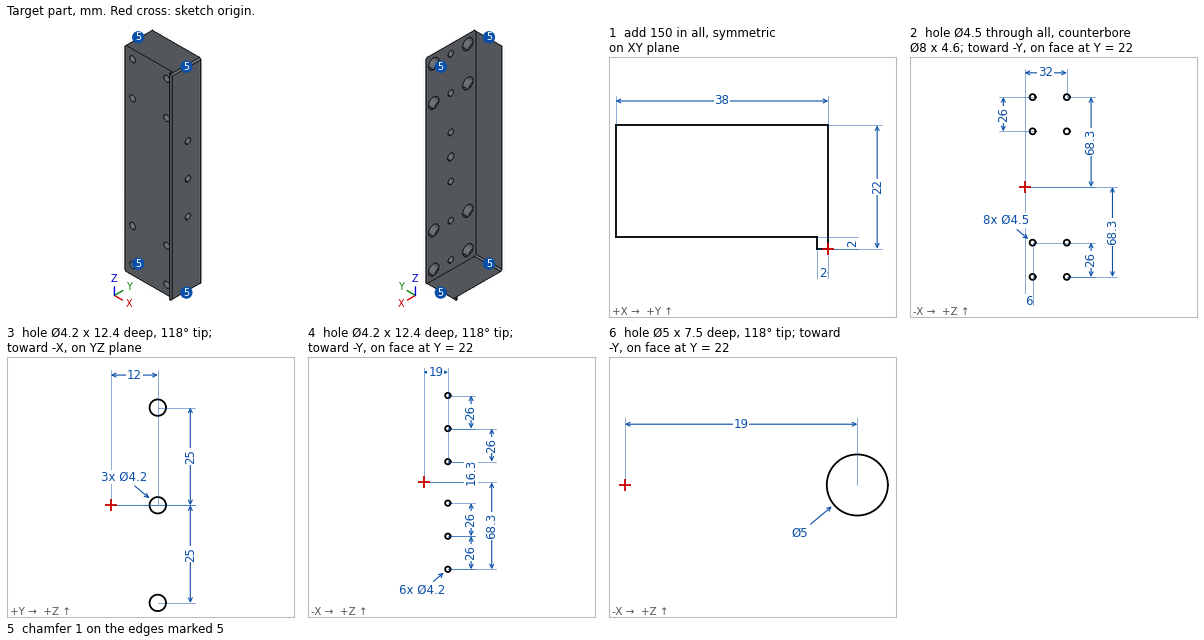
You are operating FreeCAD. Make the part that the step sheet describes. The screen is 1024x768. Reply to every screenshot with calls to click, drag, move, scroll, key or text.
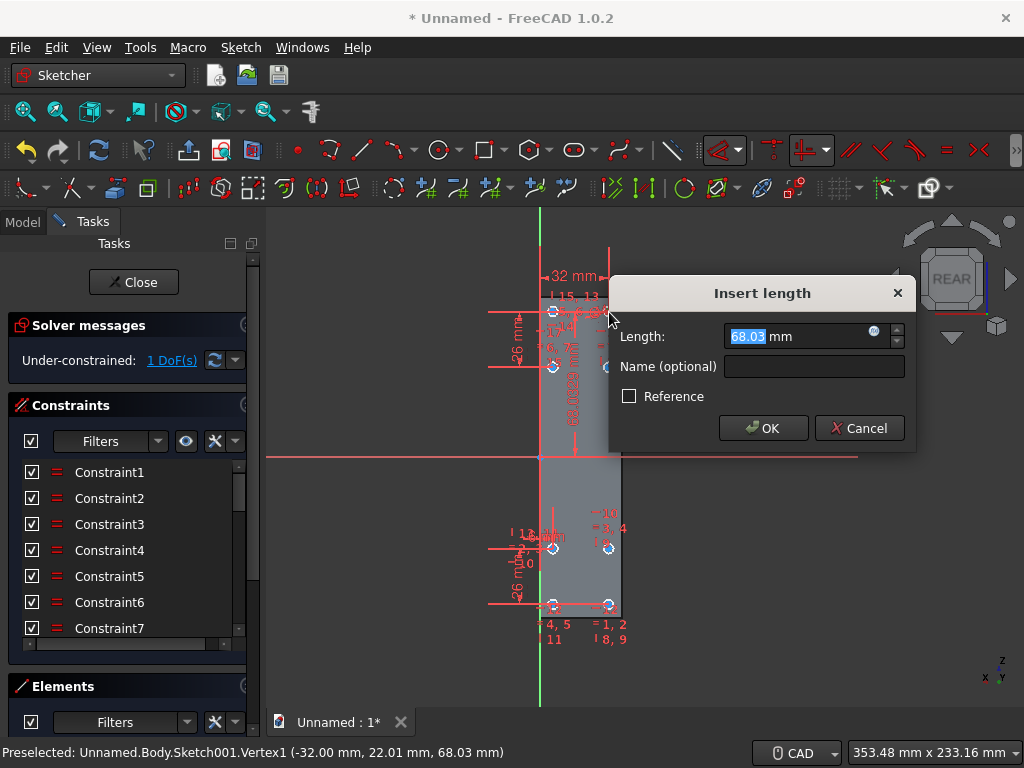
text(68.3)
key(Return)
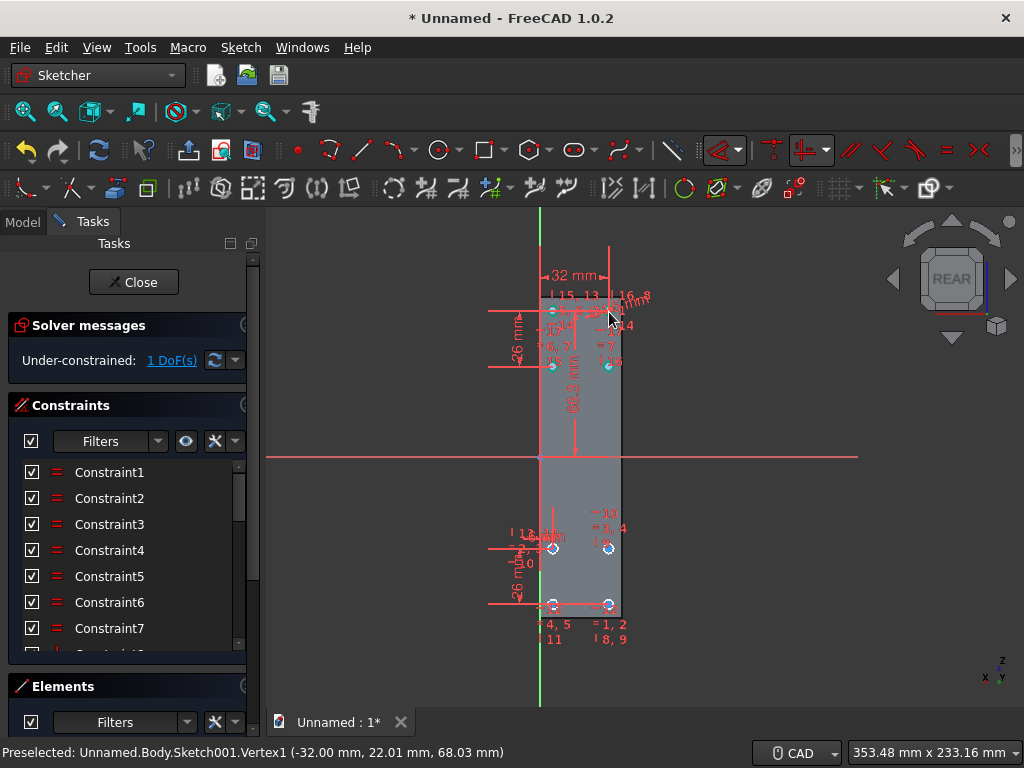
click(609, 604)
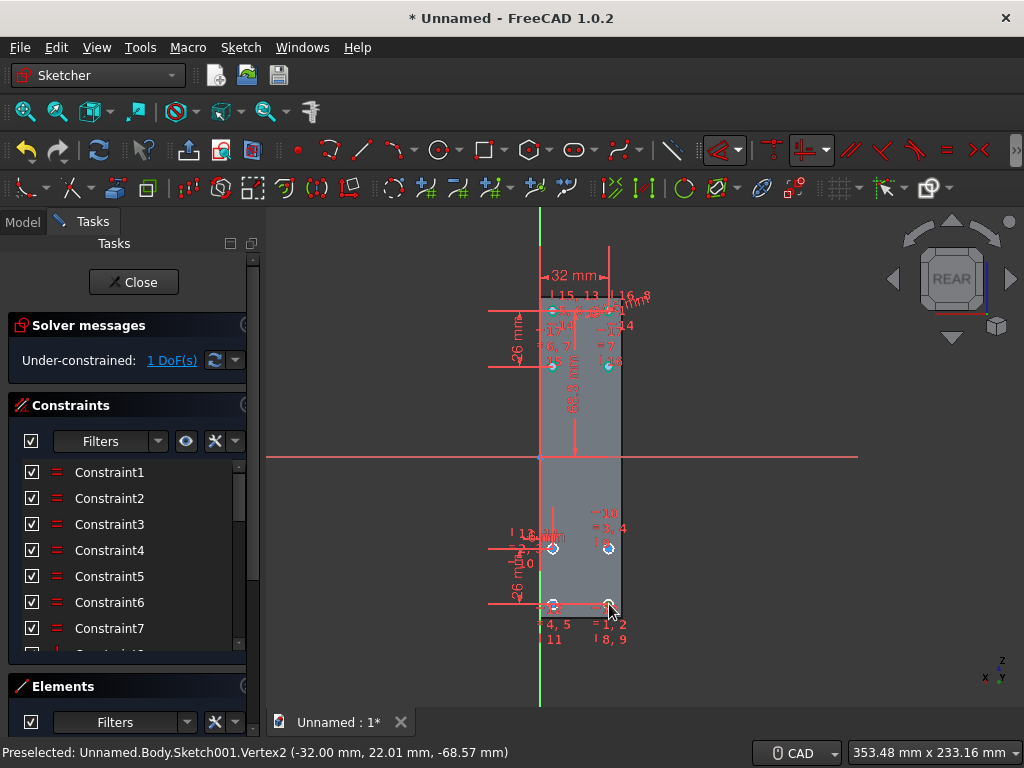
key(i)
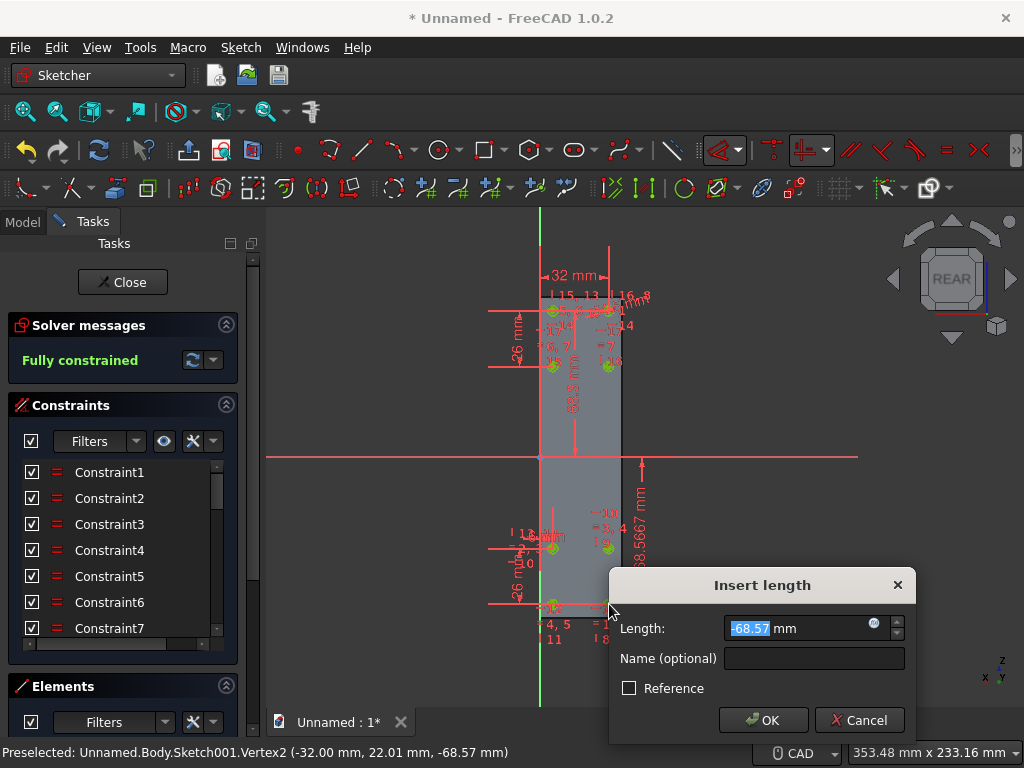
text(-68.3)
key(Return)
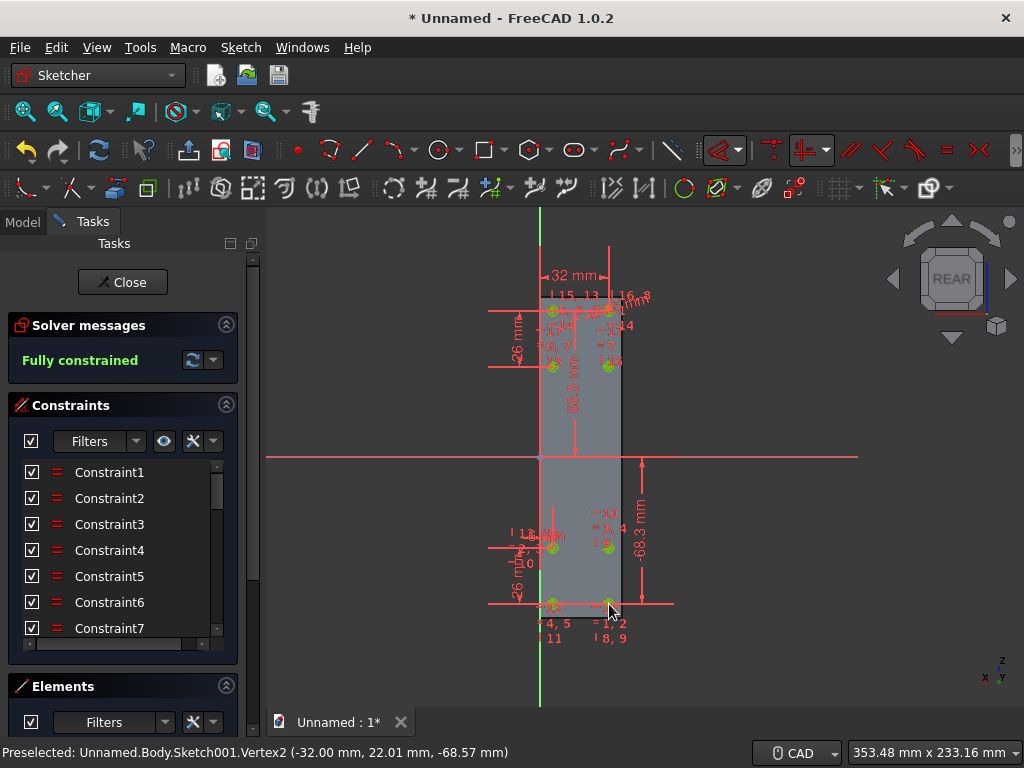
click(123, 282)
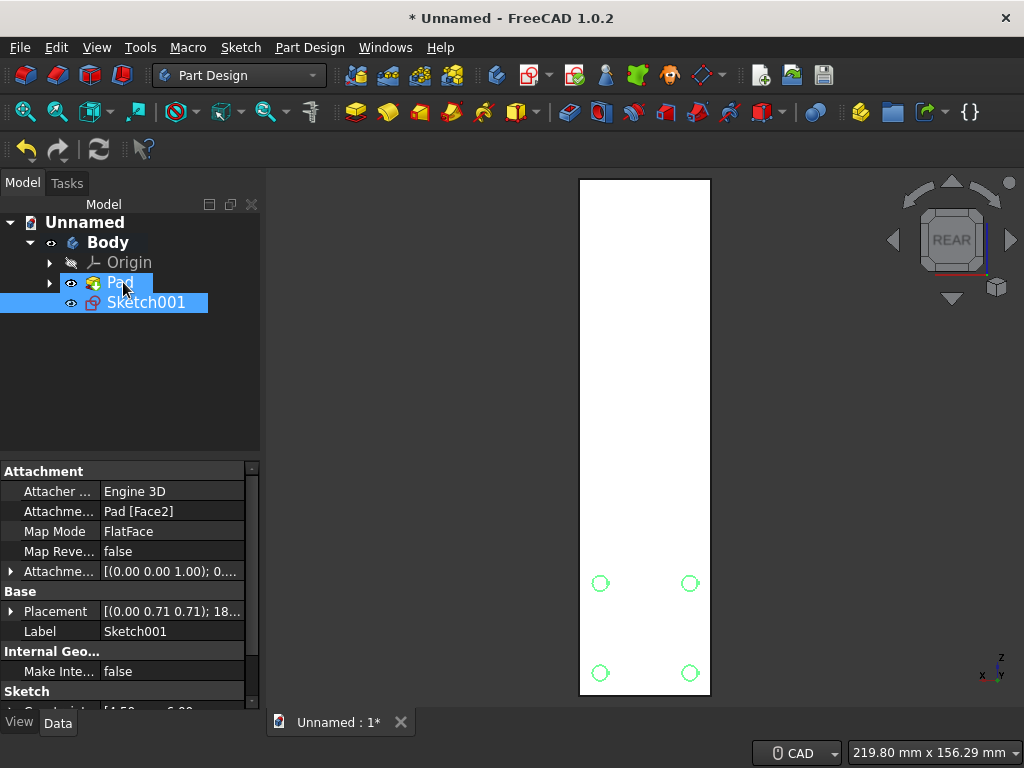
click(602, 112)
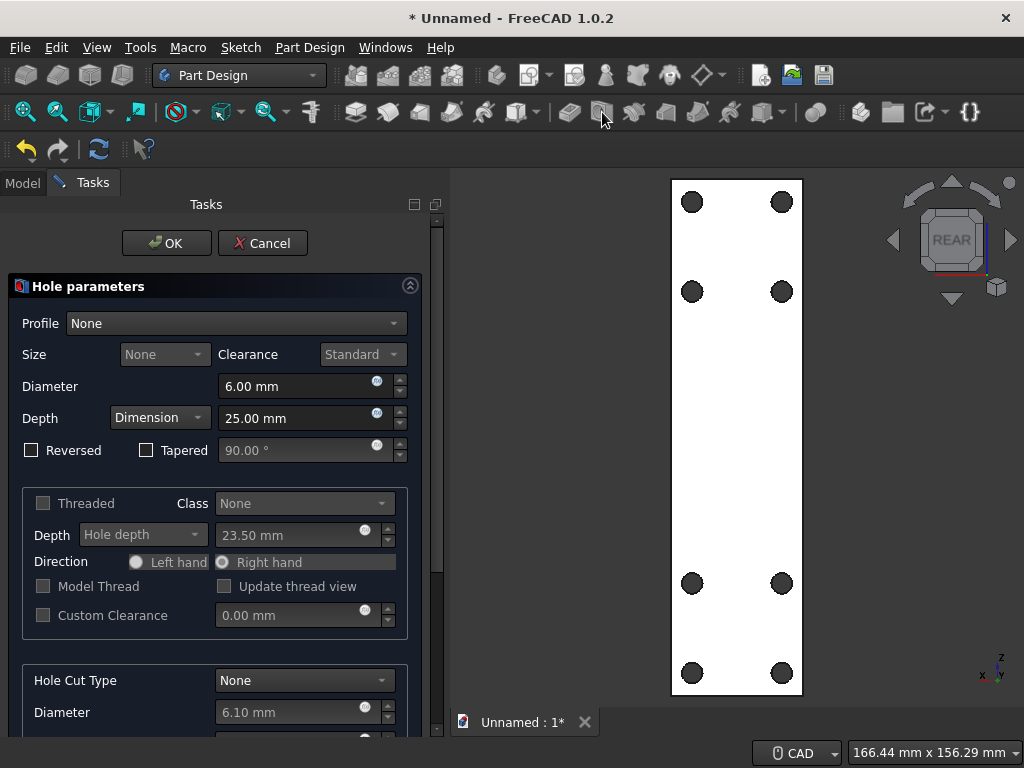
triple_click(305, 386)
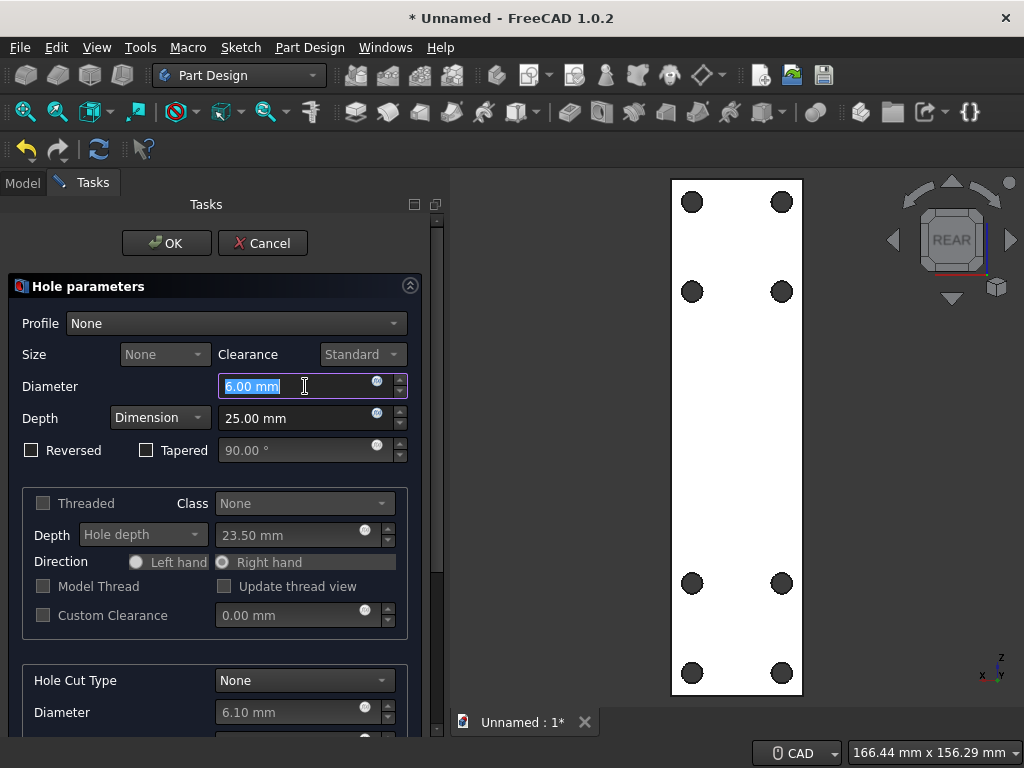
text(4.5)
key(Tab)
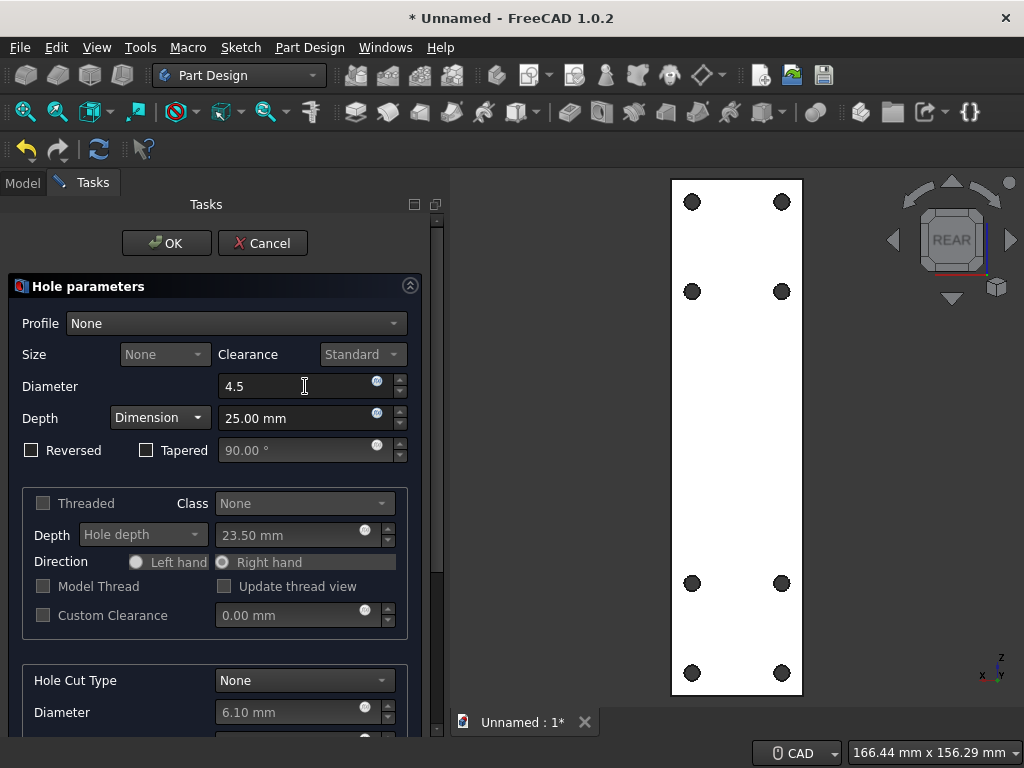
click(161, 418)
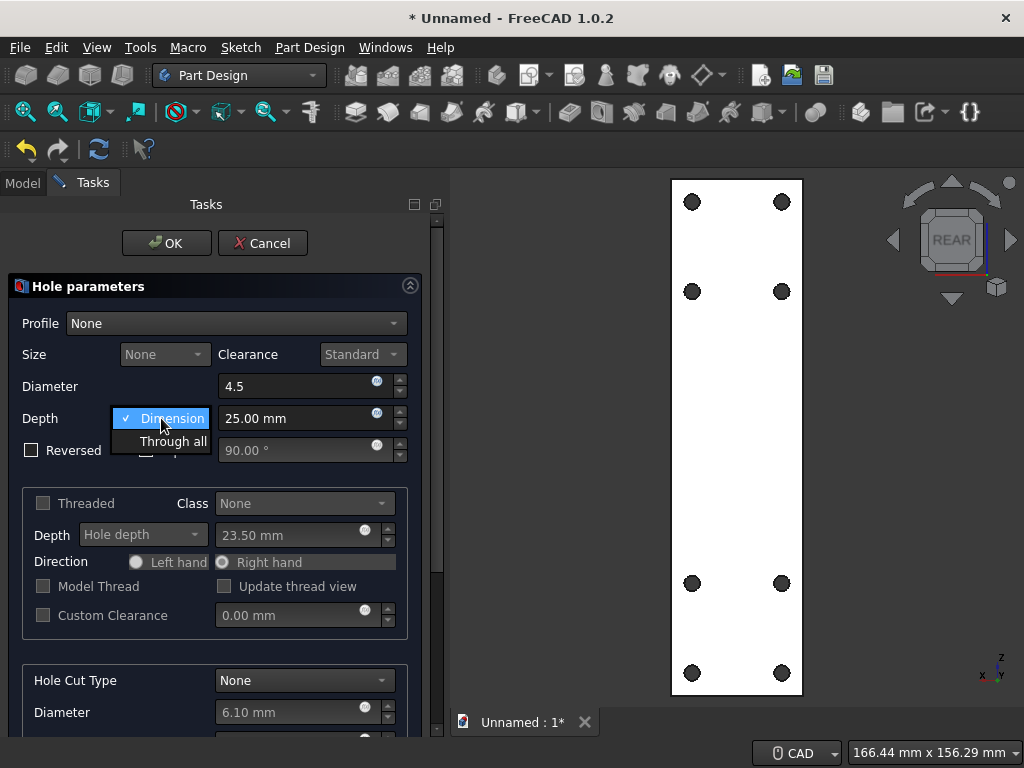
click(160, 442)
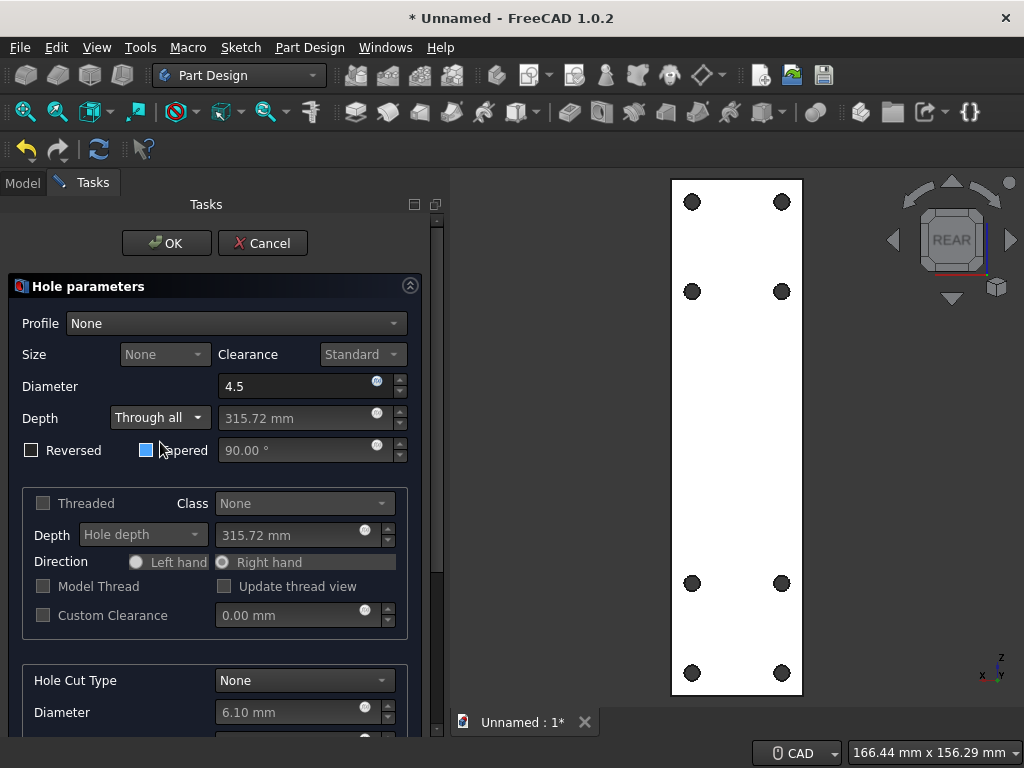
click(306, 680)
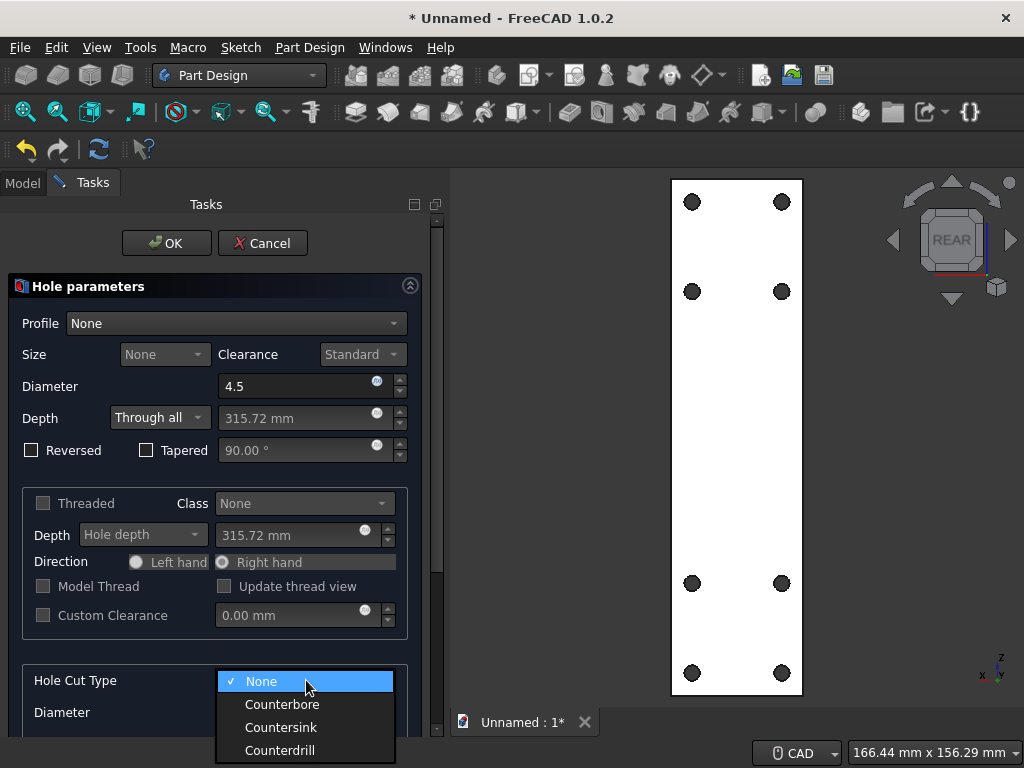
click(304, 704)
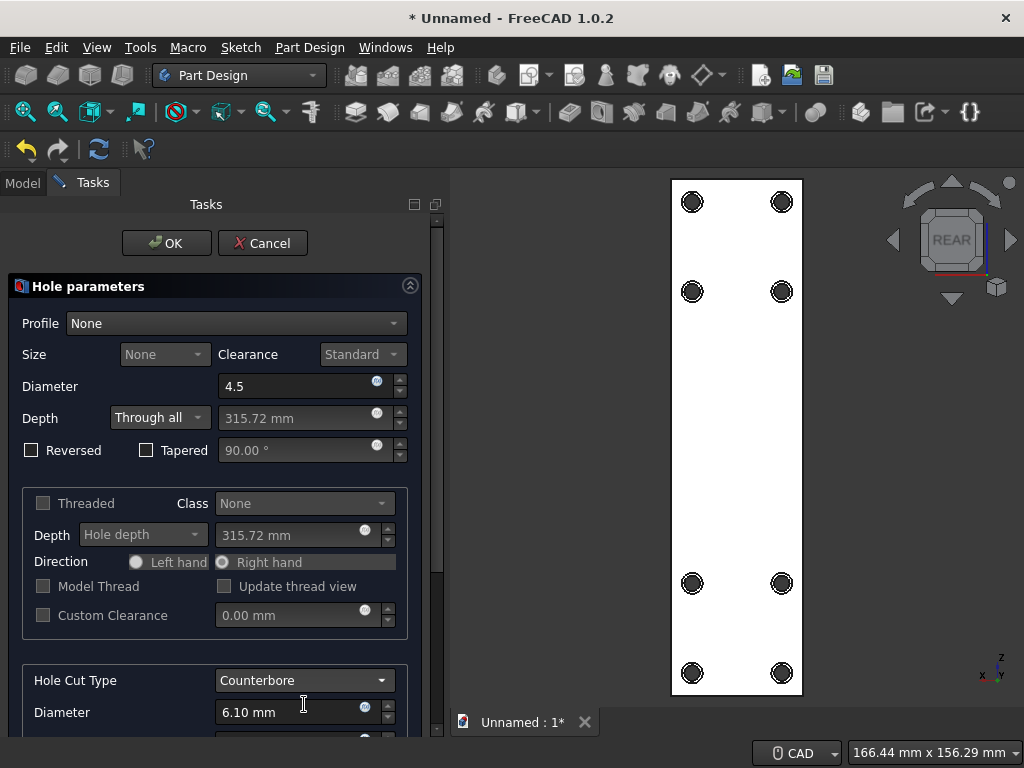
triple_click(298, 712)